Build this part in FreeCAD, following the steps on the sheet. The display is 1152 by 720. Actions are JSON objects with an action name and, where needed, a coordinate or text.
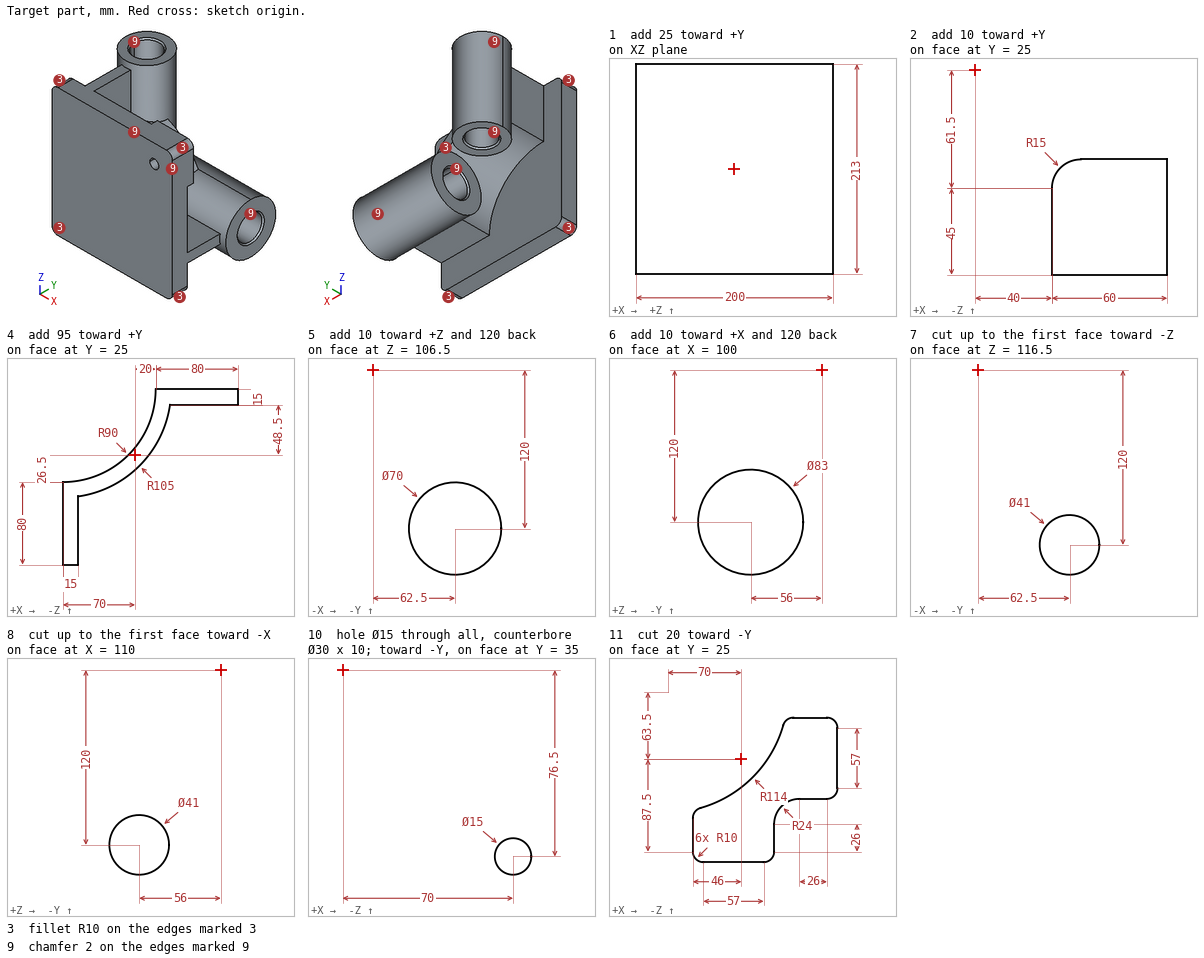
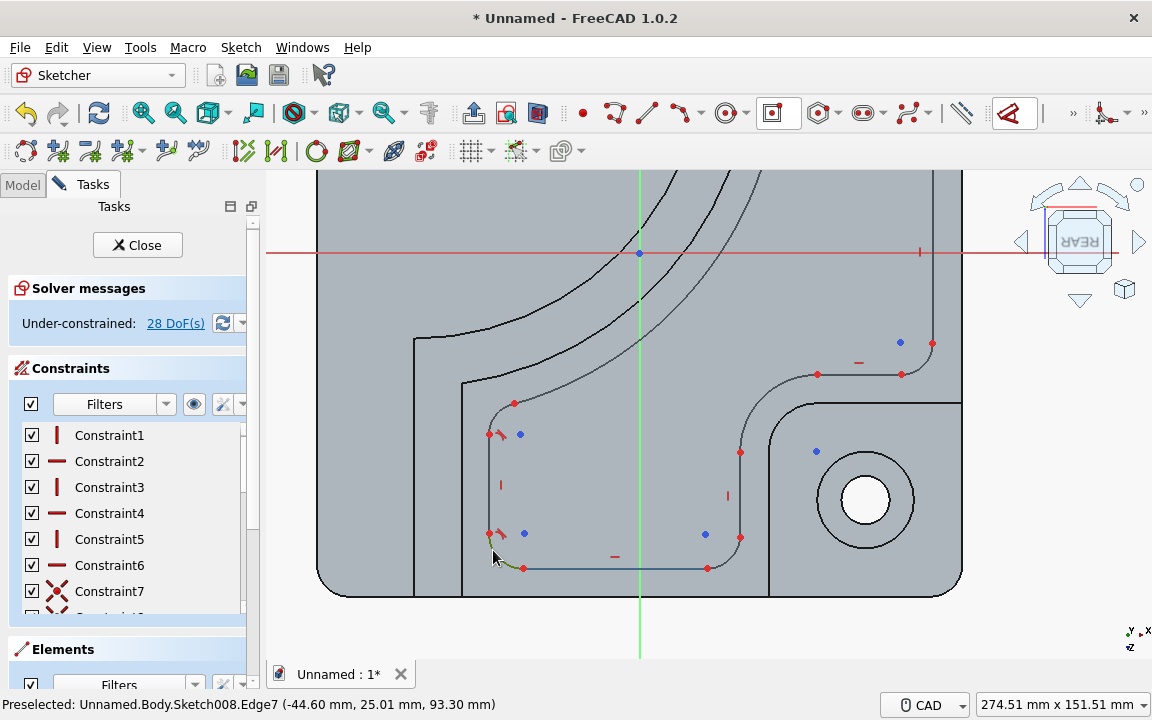
{"action": "key", "text": "t"}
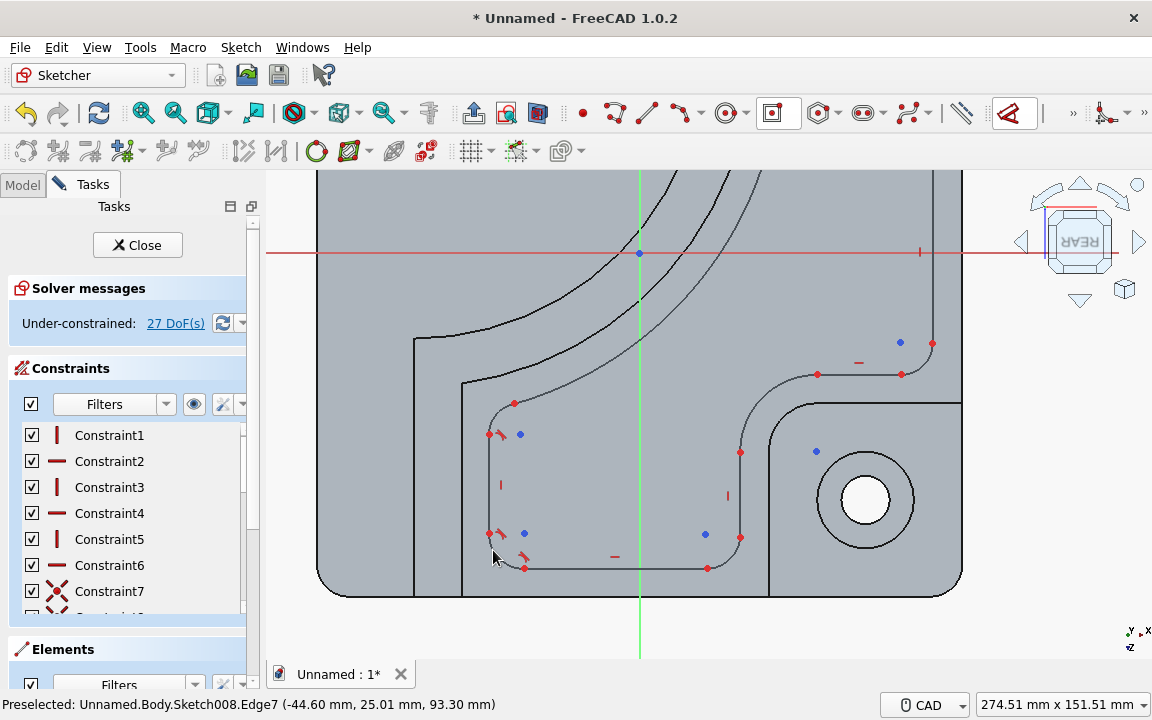
{"action": "left_click", "coordinate": [579, 569]}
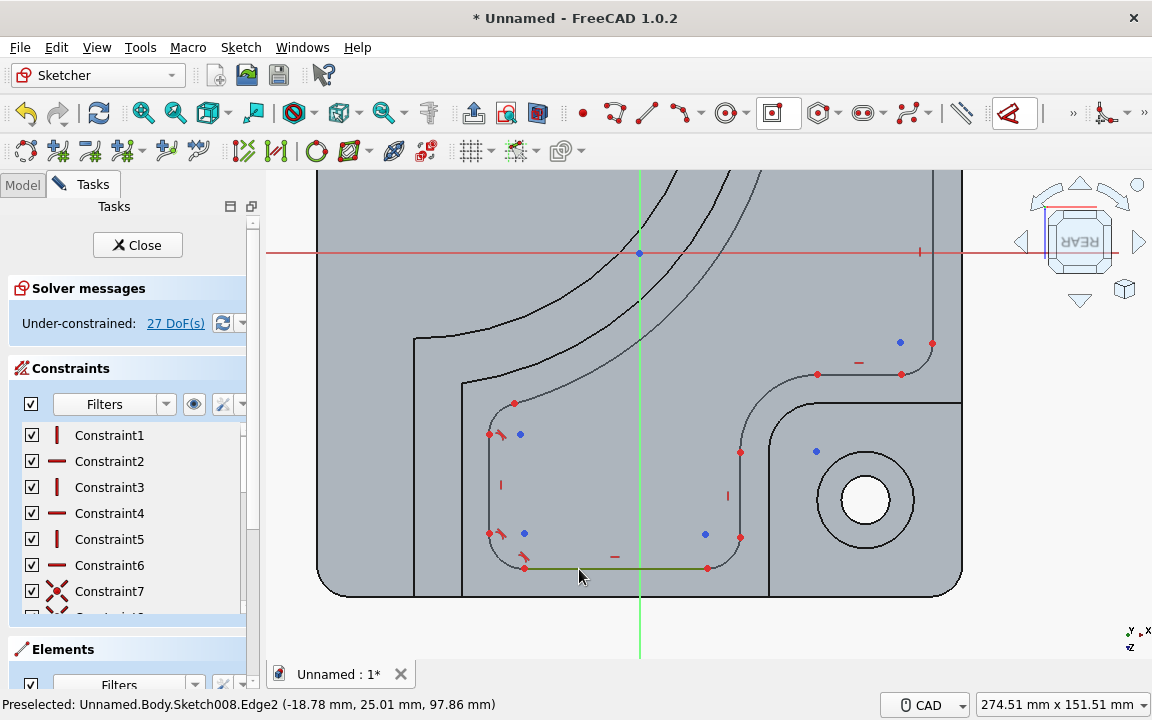
{"action": "left_click", "coordinate": [722, 565]}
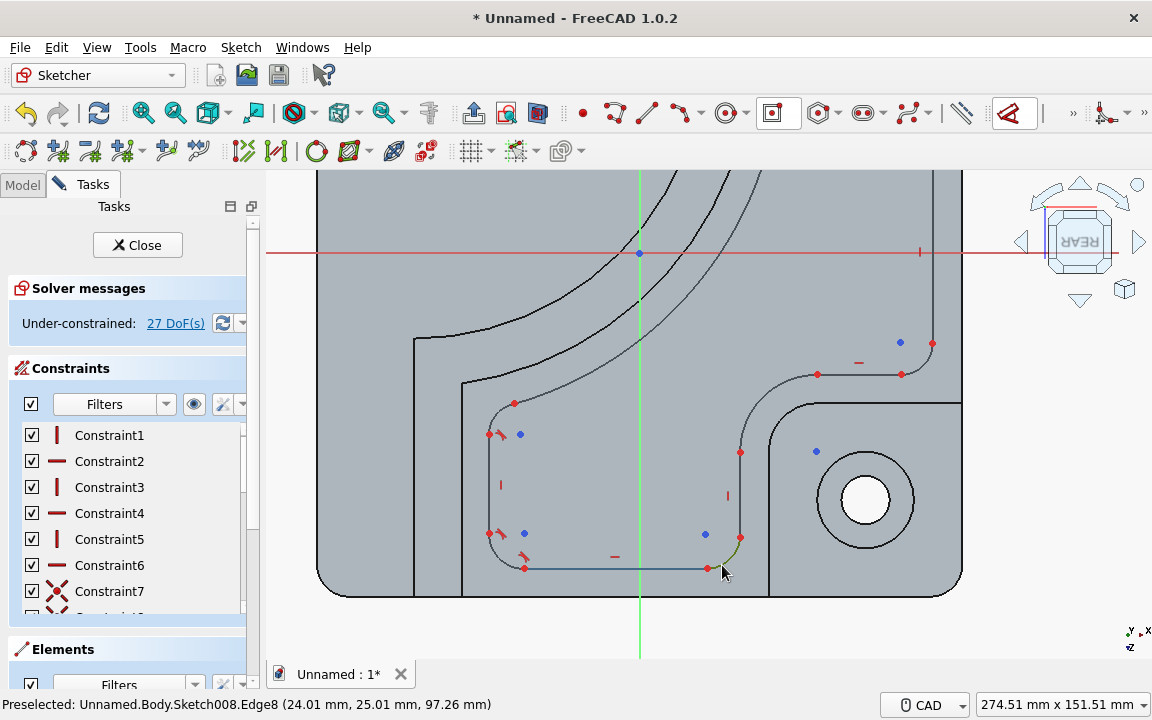
{"action": "key", "text": "t"}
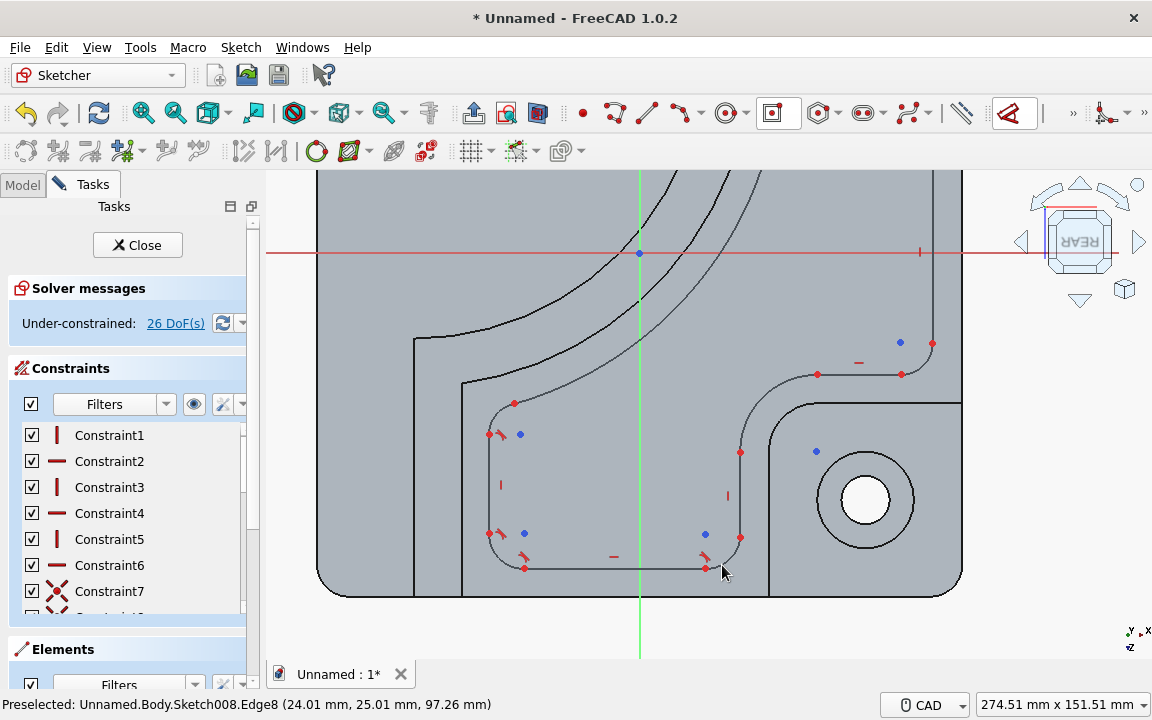
{"action": "left_click", "coordinate": [740, 512]}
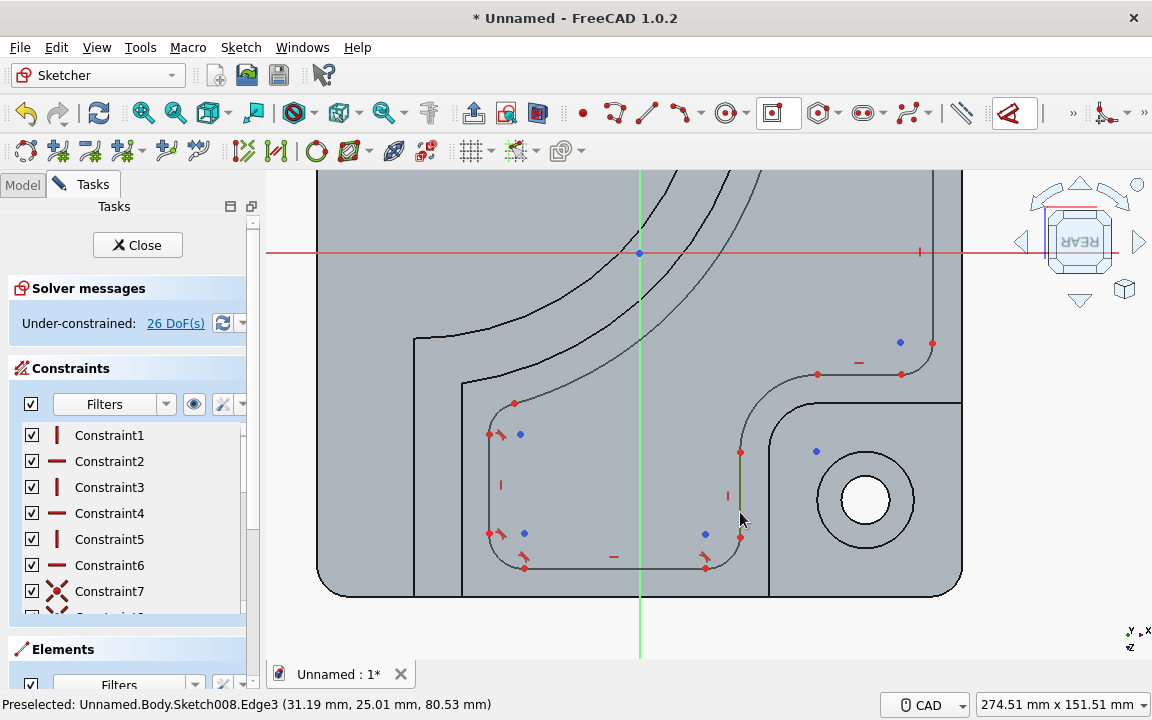
{"action": "left_click", "coordinate": [720, 566]}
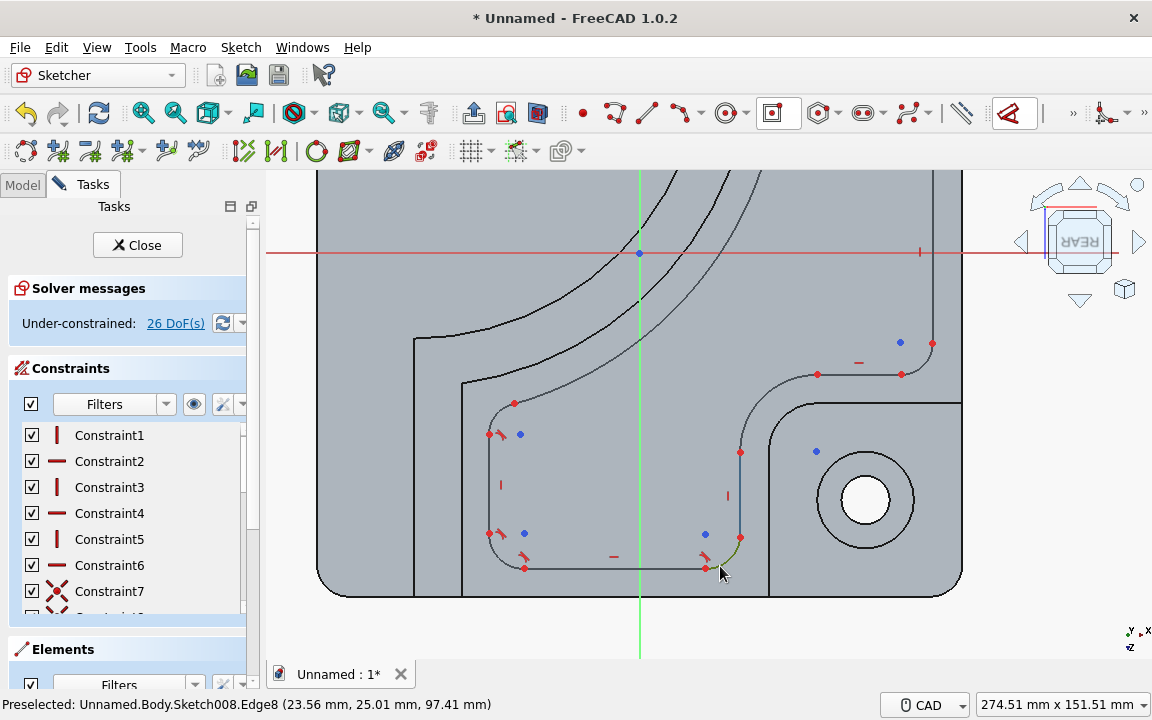
{"action": "key", "text": "t"}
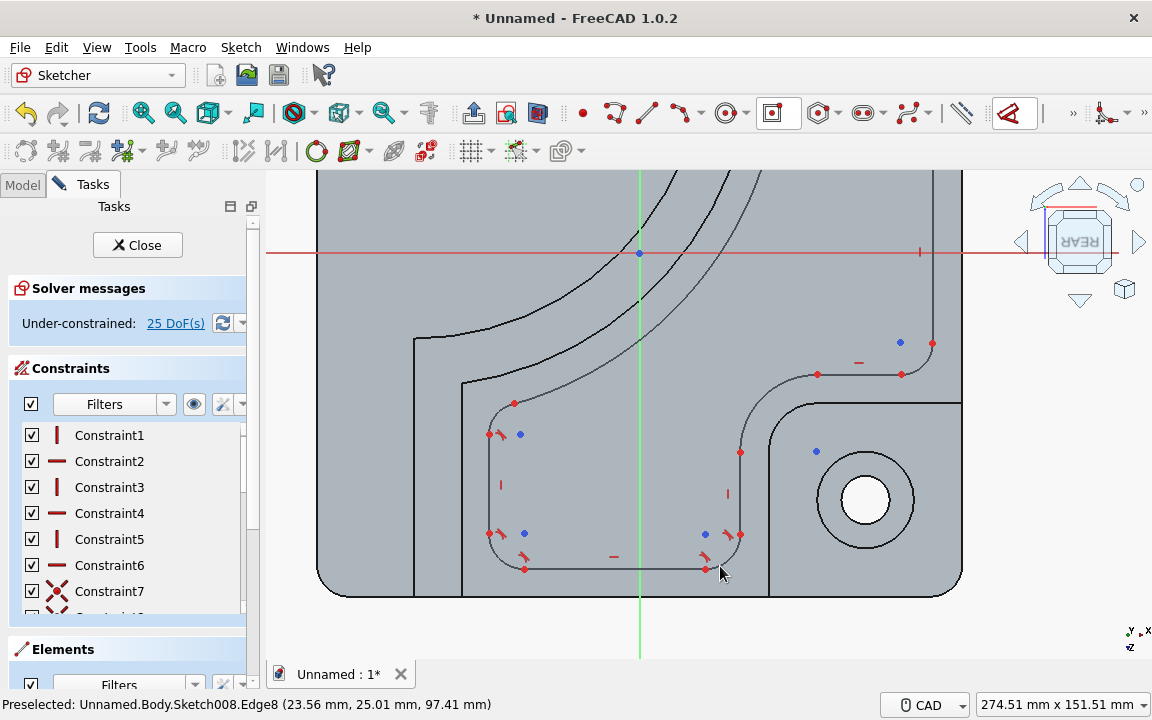
{"action": "left_click", "coordinate": [740, 510]}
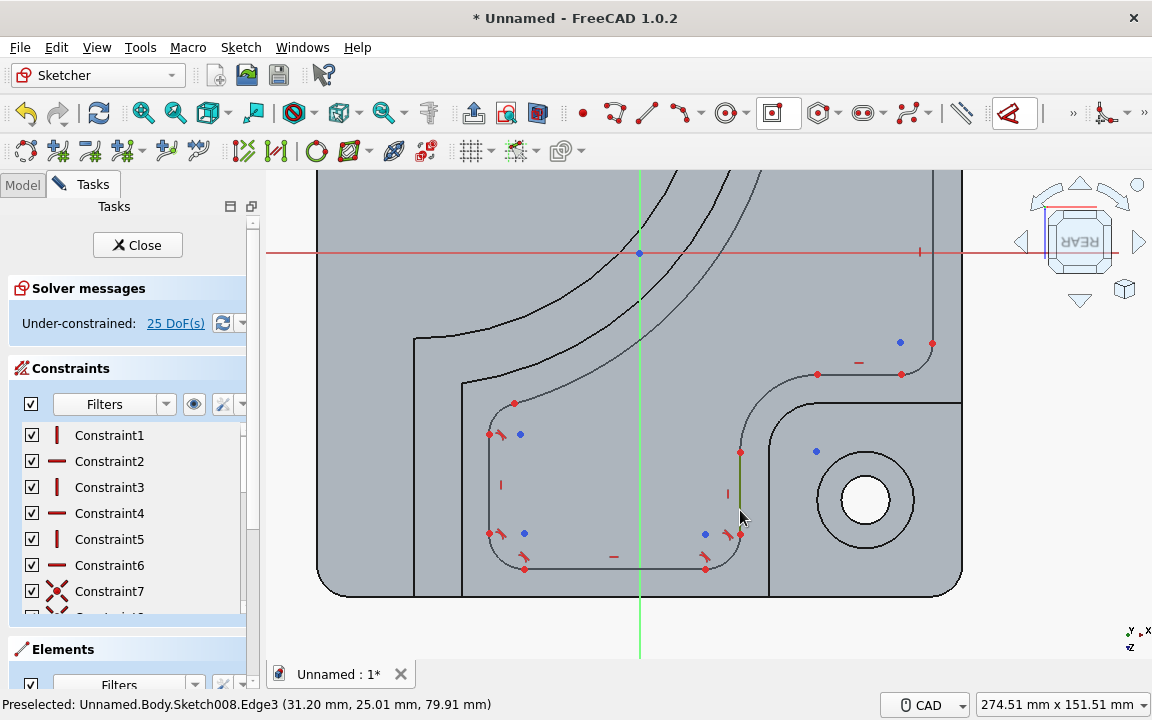
{"action": "left_click", "coordinate": [782, 383]}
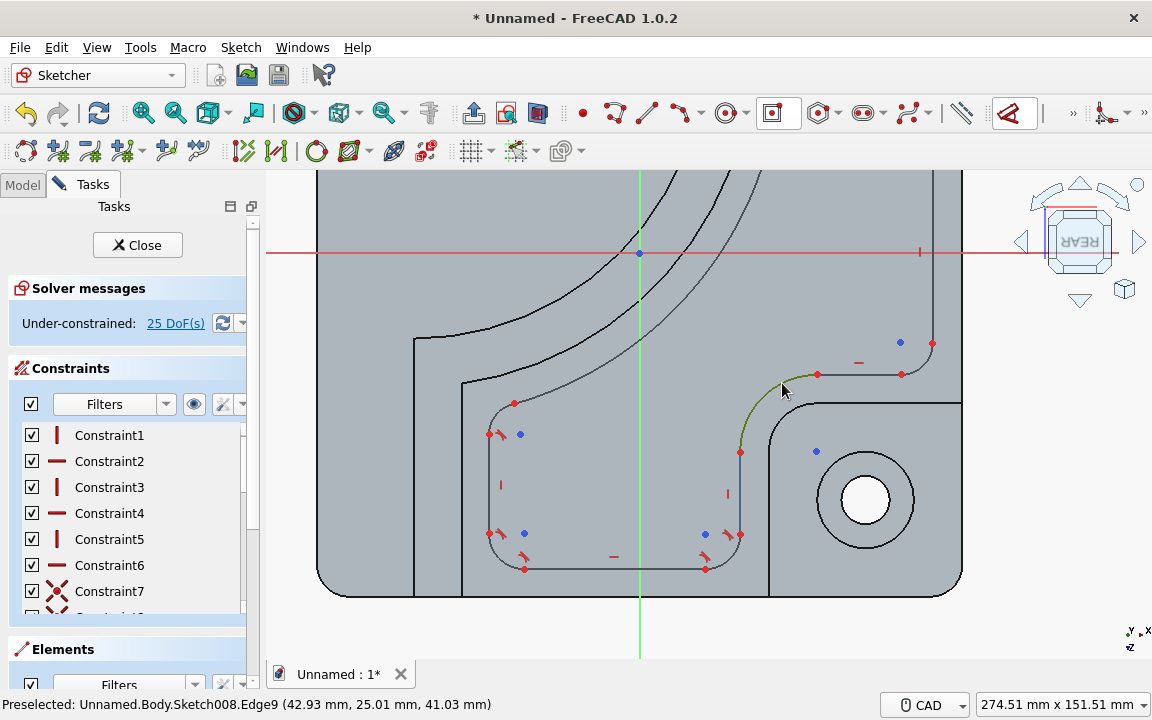
{"action": "key", "text": "t"}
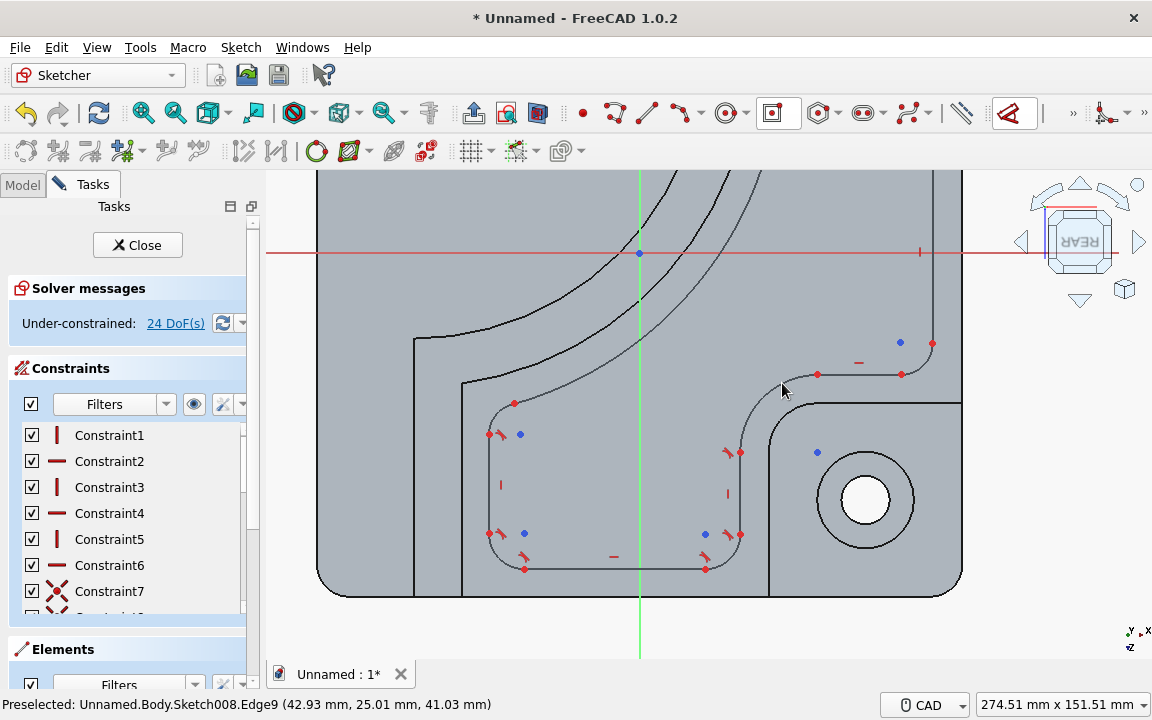
{"action": "left_click", "coordinate": [843, 375]}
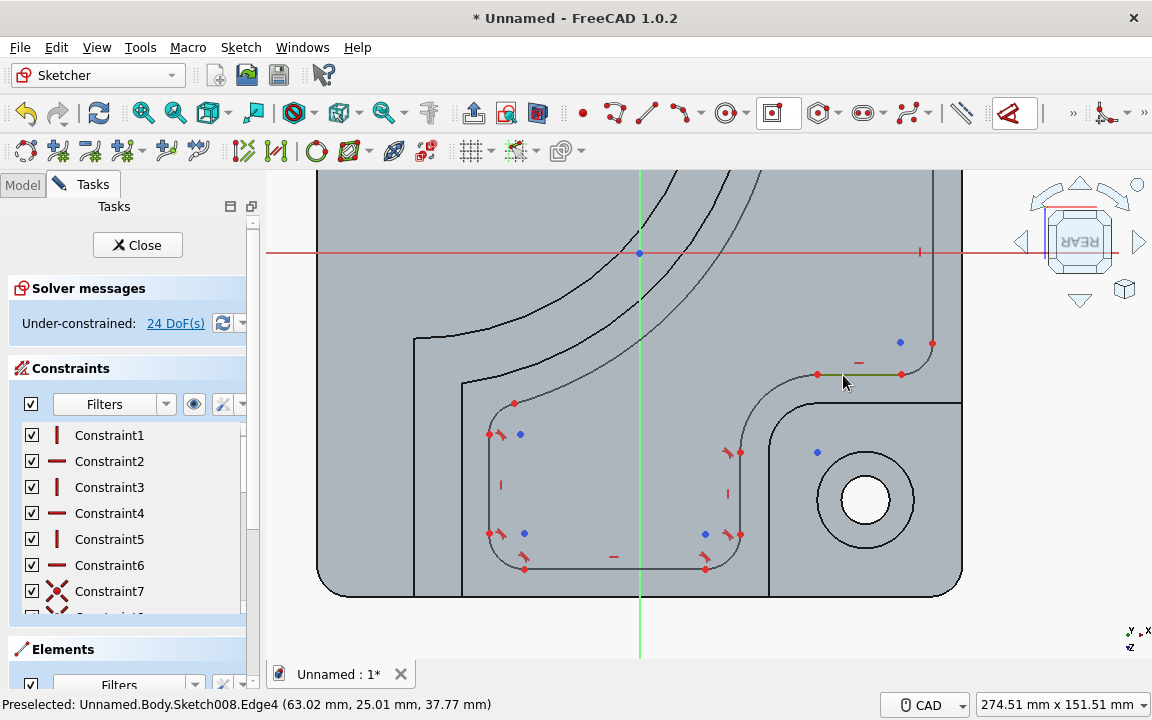
{"action": "left_click", "coordinate": [783, 383]}